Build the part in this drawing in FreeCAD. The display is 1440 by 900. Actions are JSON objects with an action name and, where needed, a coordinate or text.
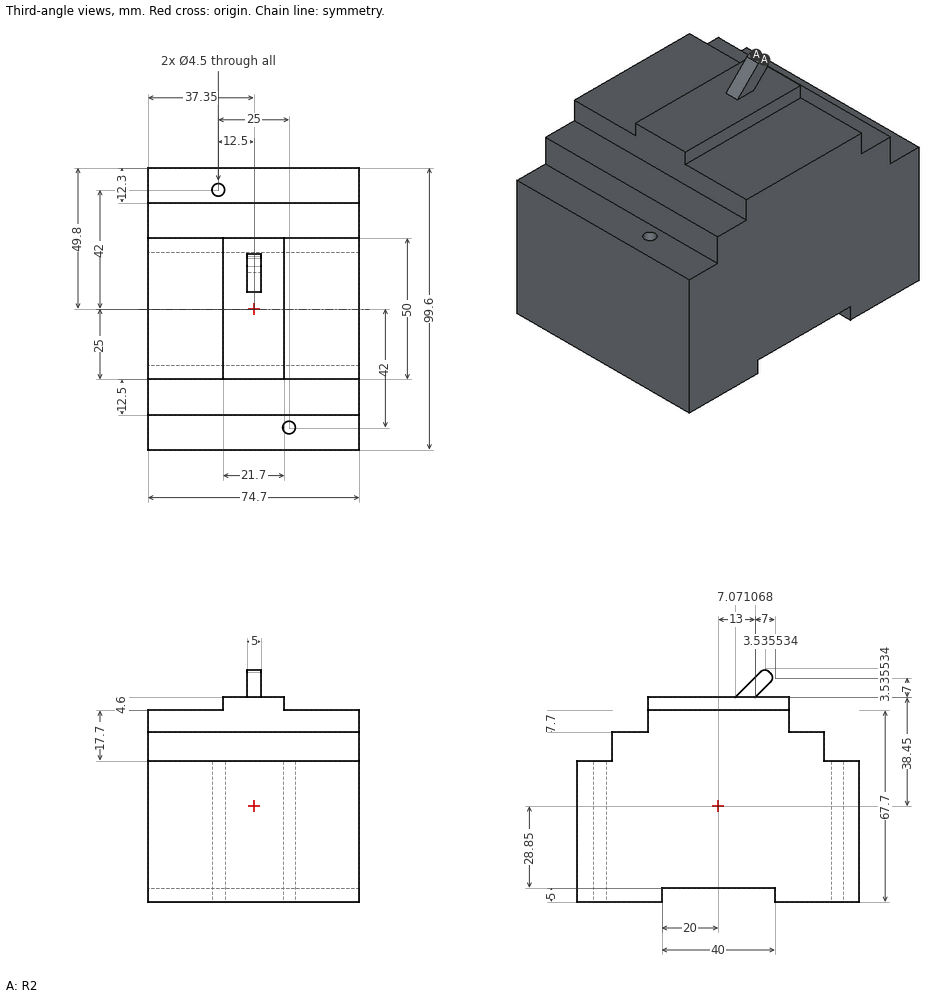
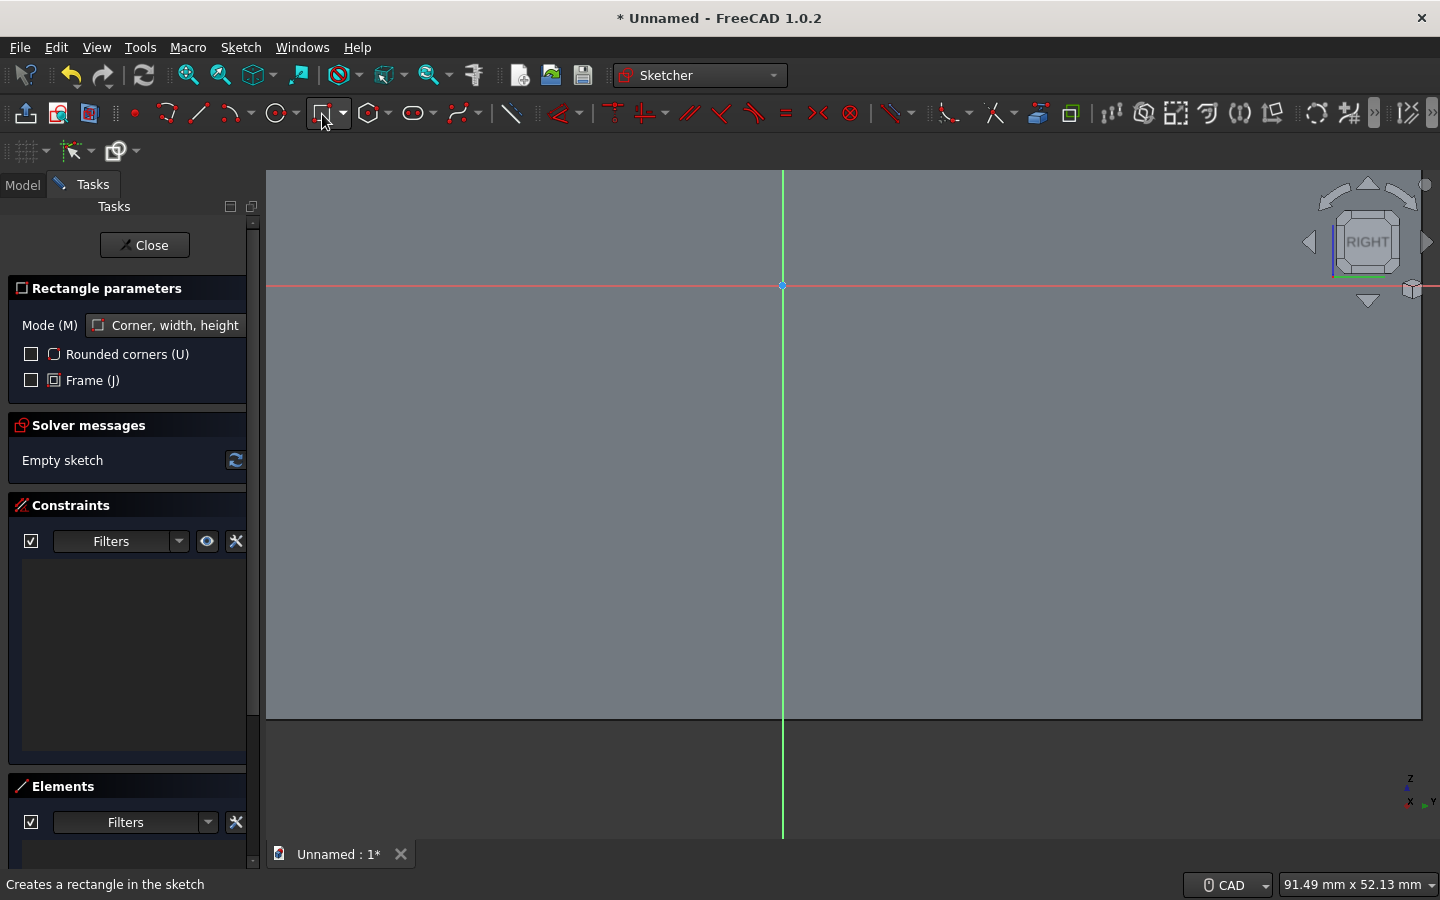
{"action": "left_click", "coordinate": [526, 656]}
{"action": "left_click", "coordinate": [1039, 720]}
{"action": "key", "text": "Escape"}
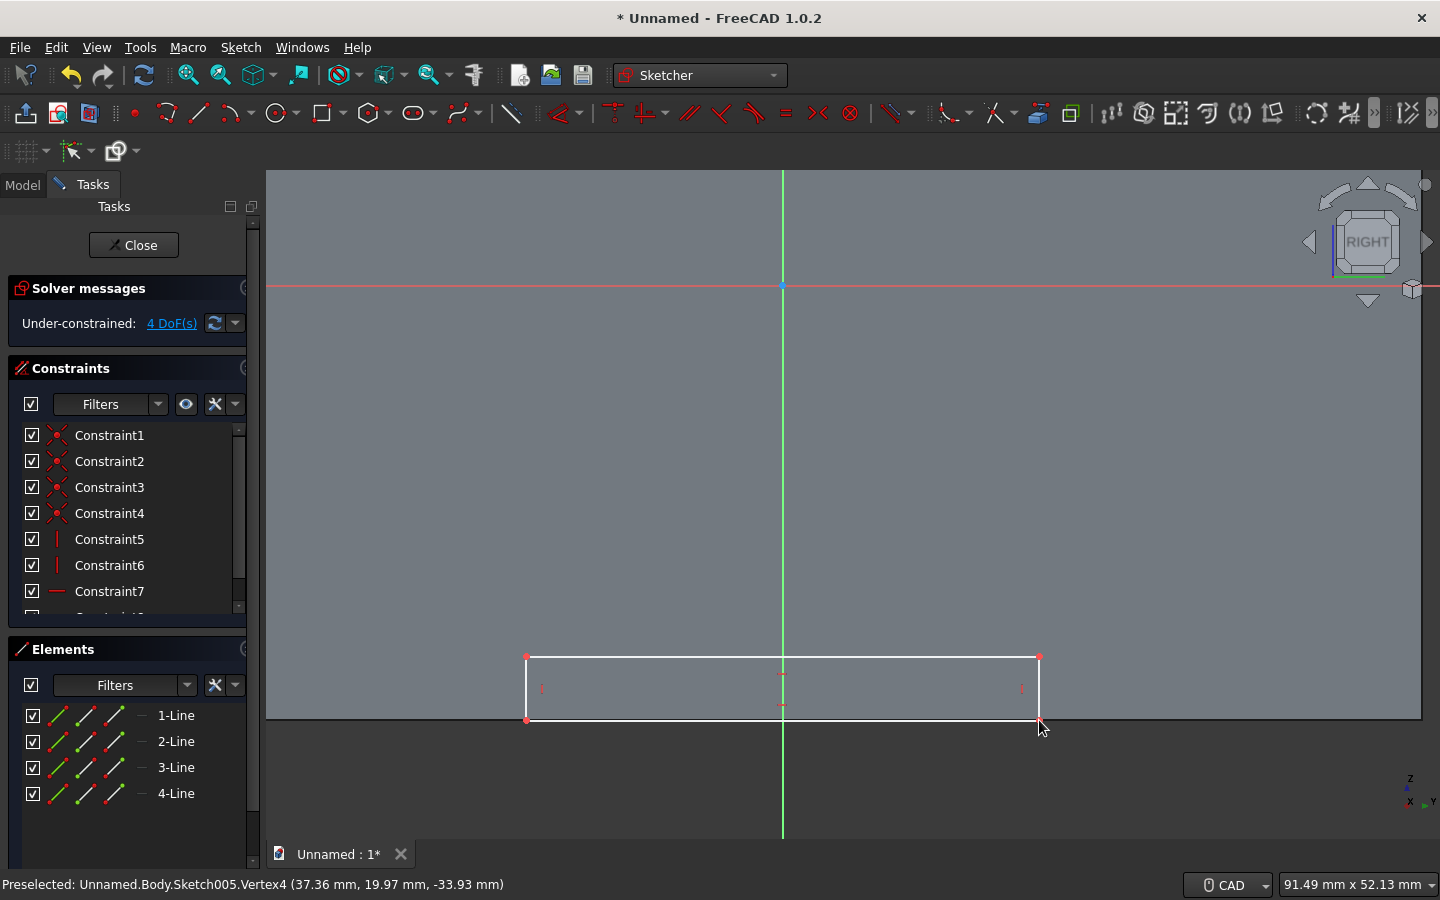
{"action": "left_click", "coordinate": [558, 114]}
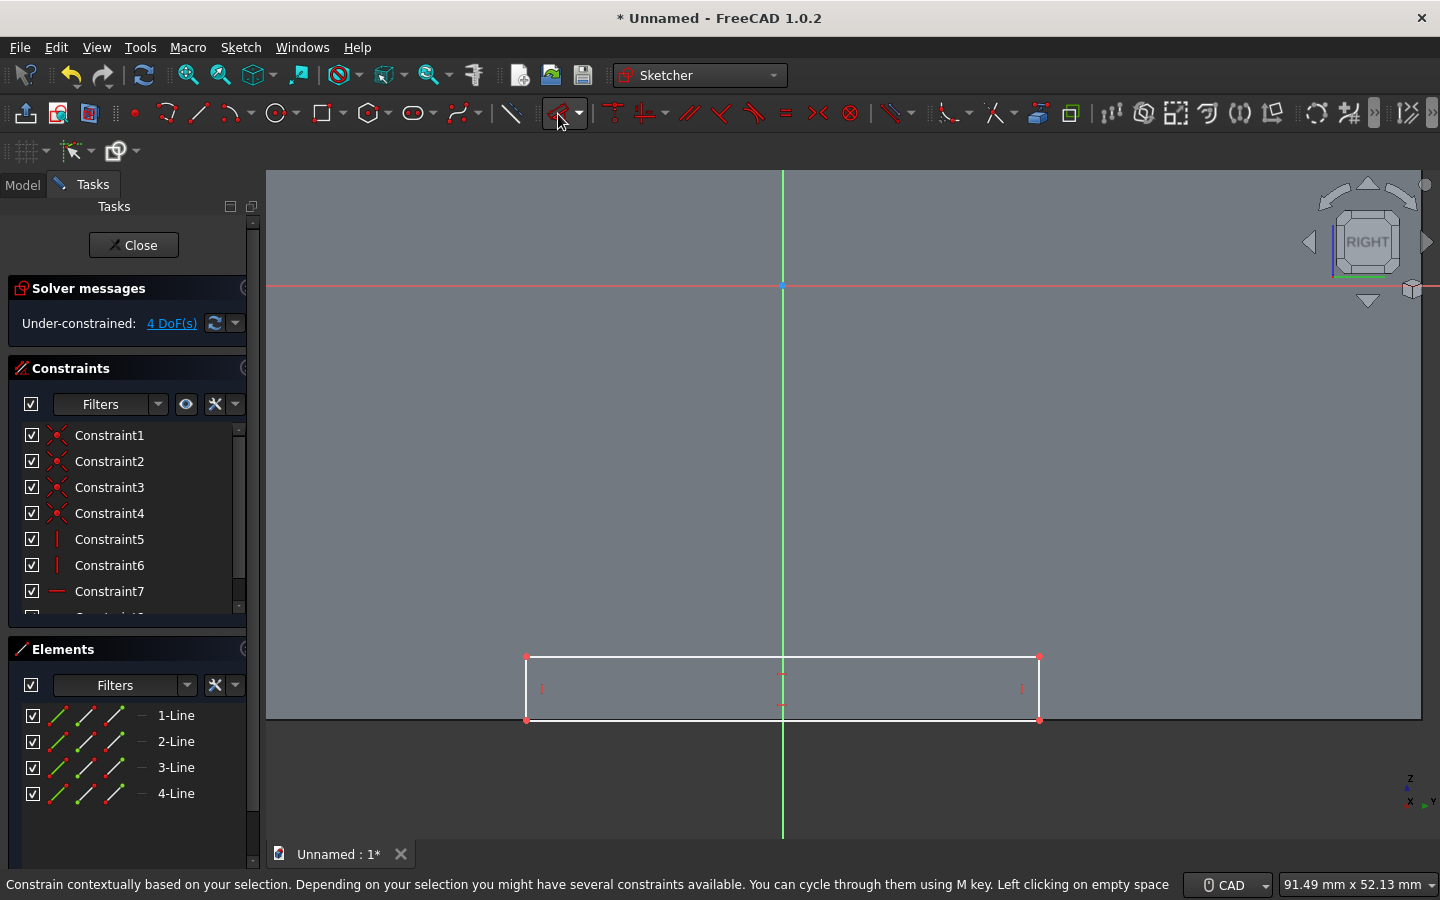
{"action": "left_click", "coordinate": [526, 676]}
{"action": "left_click", "coordinate": [492, 689]}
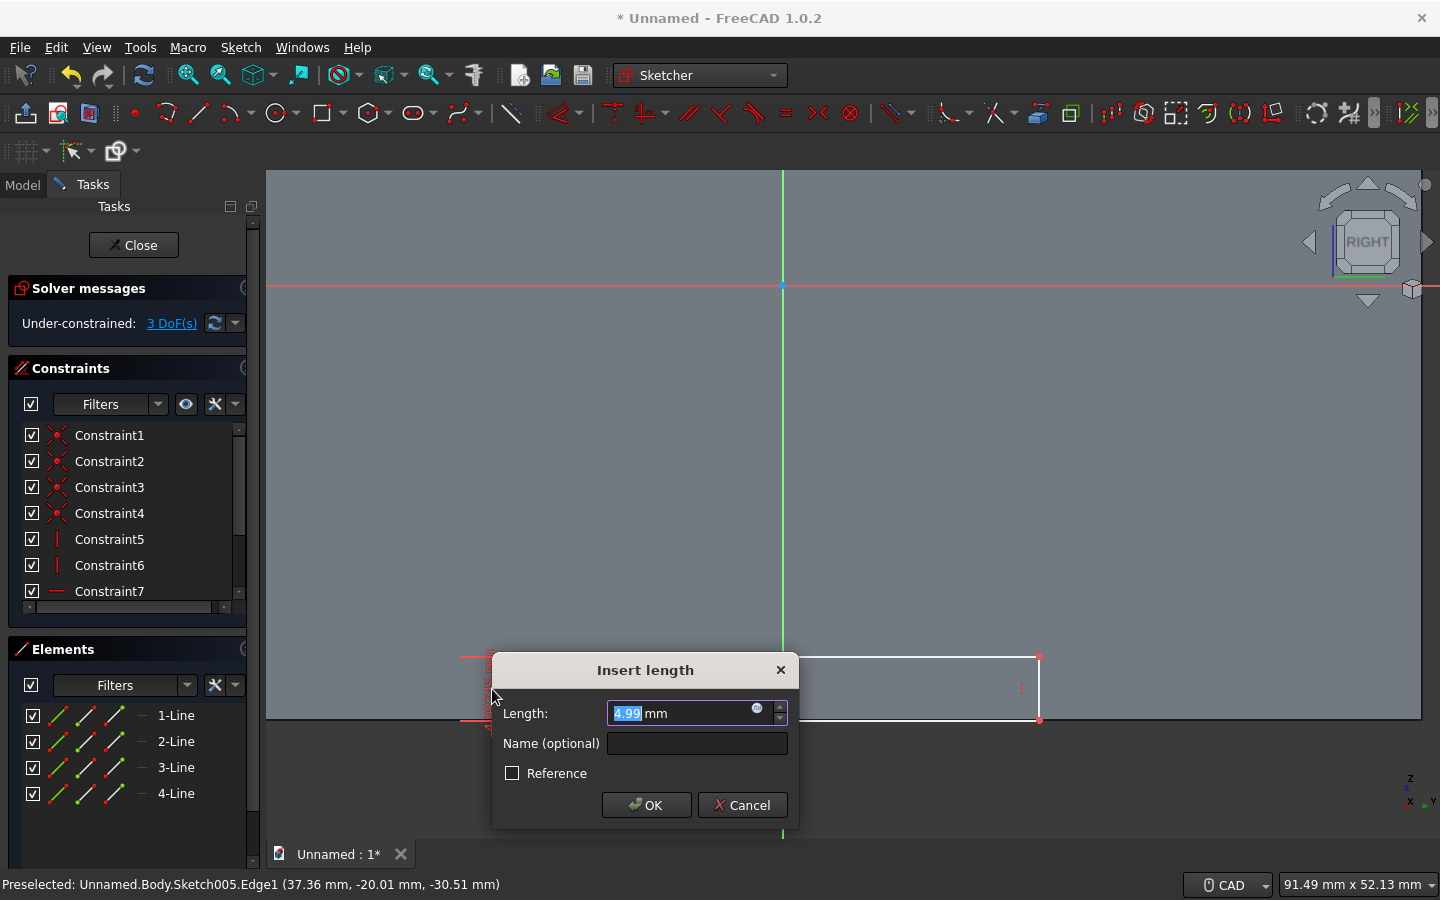
{"action": "type", "text": "5"}
{"action": "key", "text": "Return"}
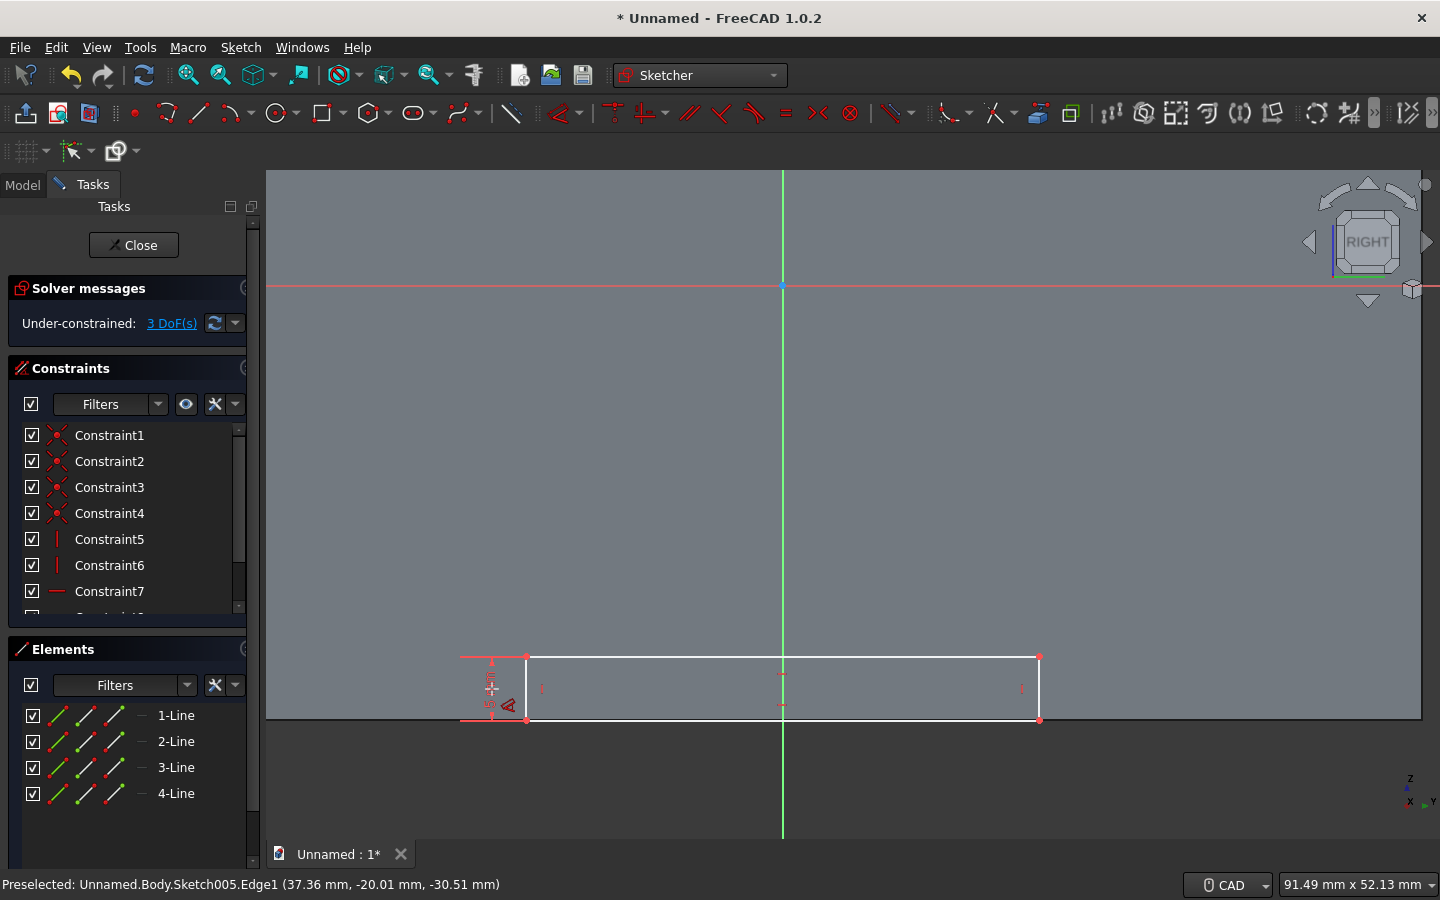
{"action": "left_click", "coordinate": [680, 721]}
{"action": "left_click", "coordinate": [665, 755]}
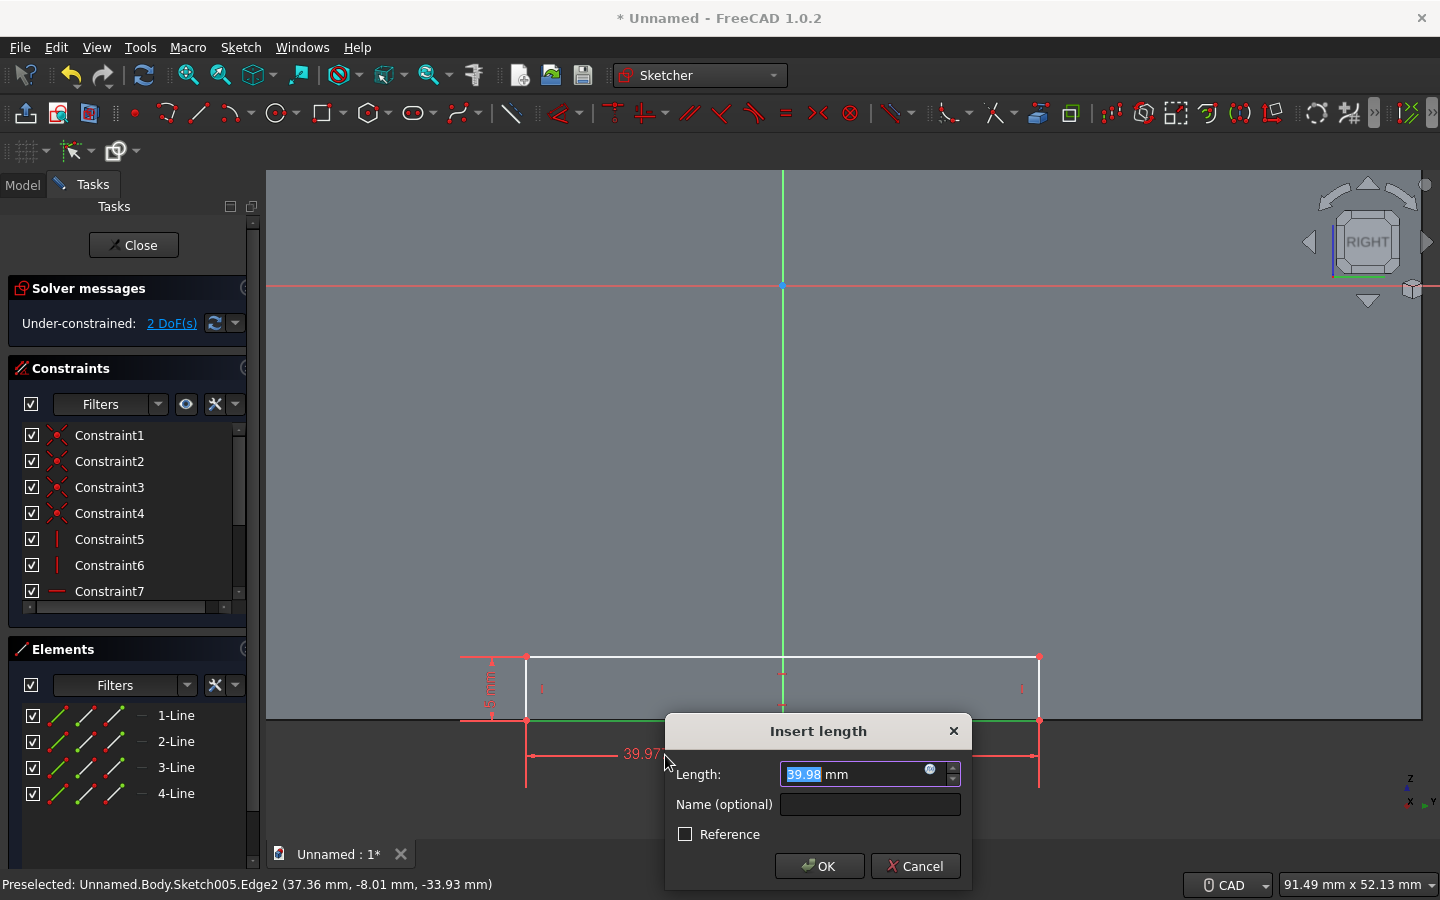
{"action": "type", "text": "40"}
{"action": "key", "text": "Return"}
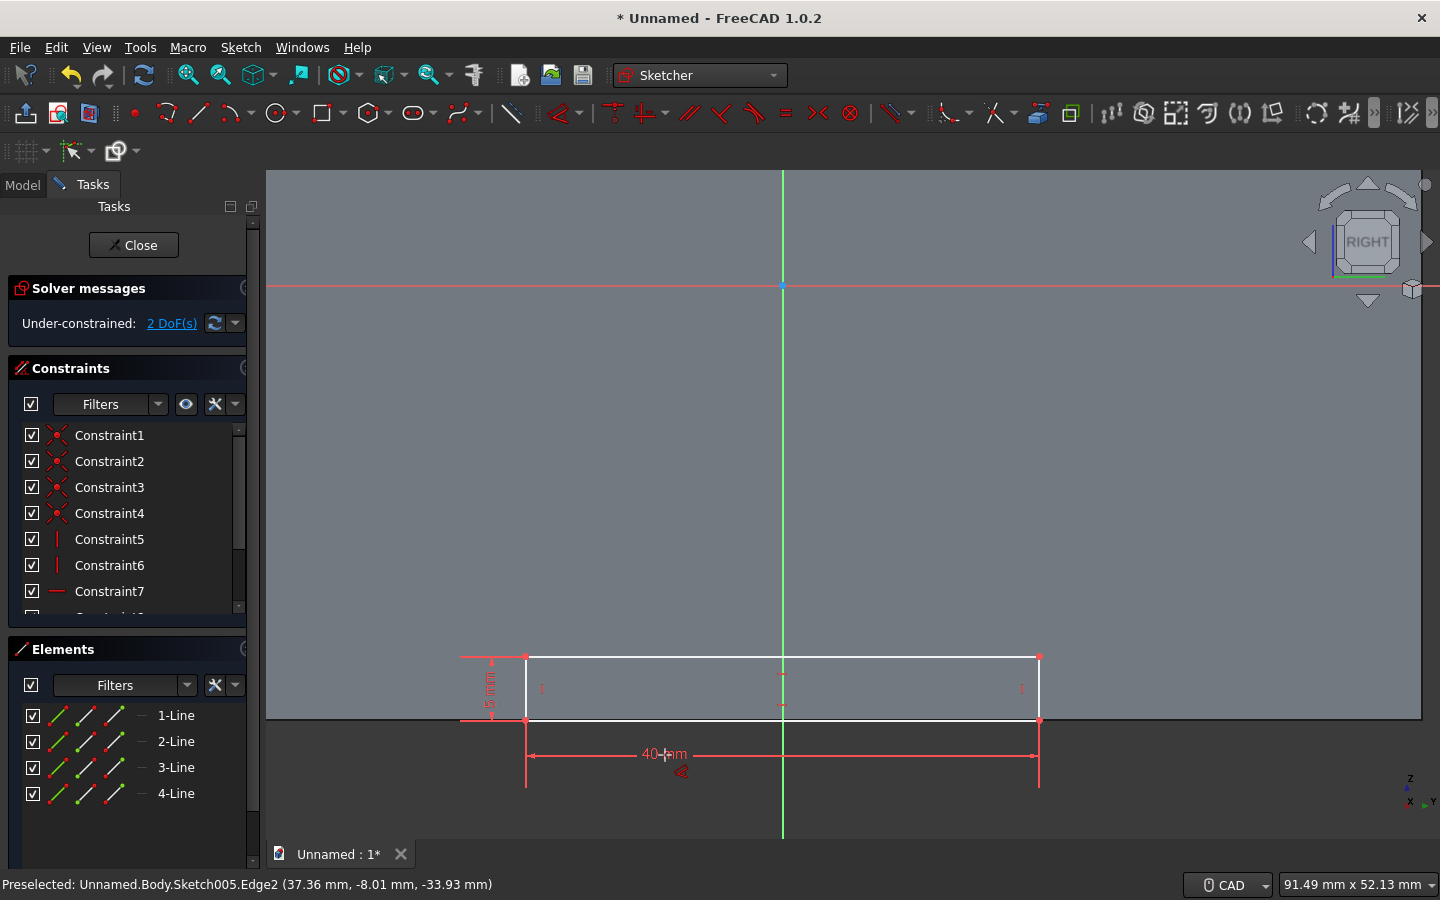
{"action": "left_click", "coordinate": [526, 657]}
{"action": "left_click", "coordinate": [654, 252]}